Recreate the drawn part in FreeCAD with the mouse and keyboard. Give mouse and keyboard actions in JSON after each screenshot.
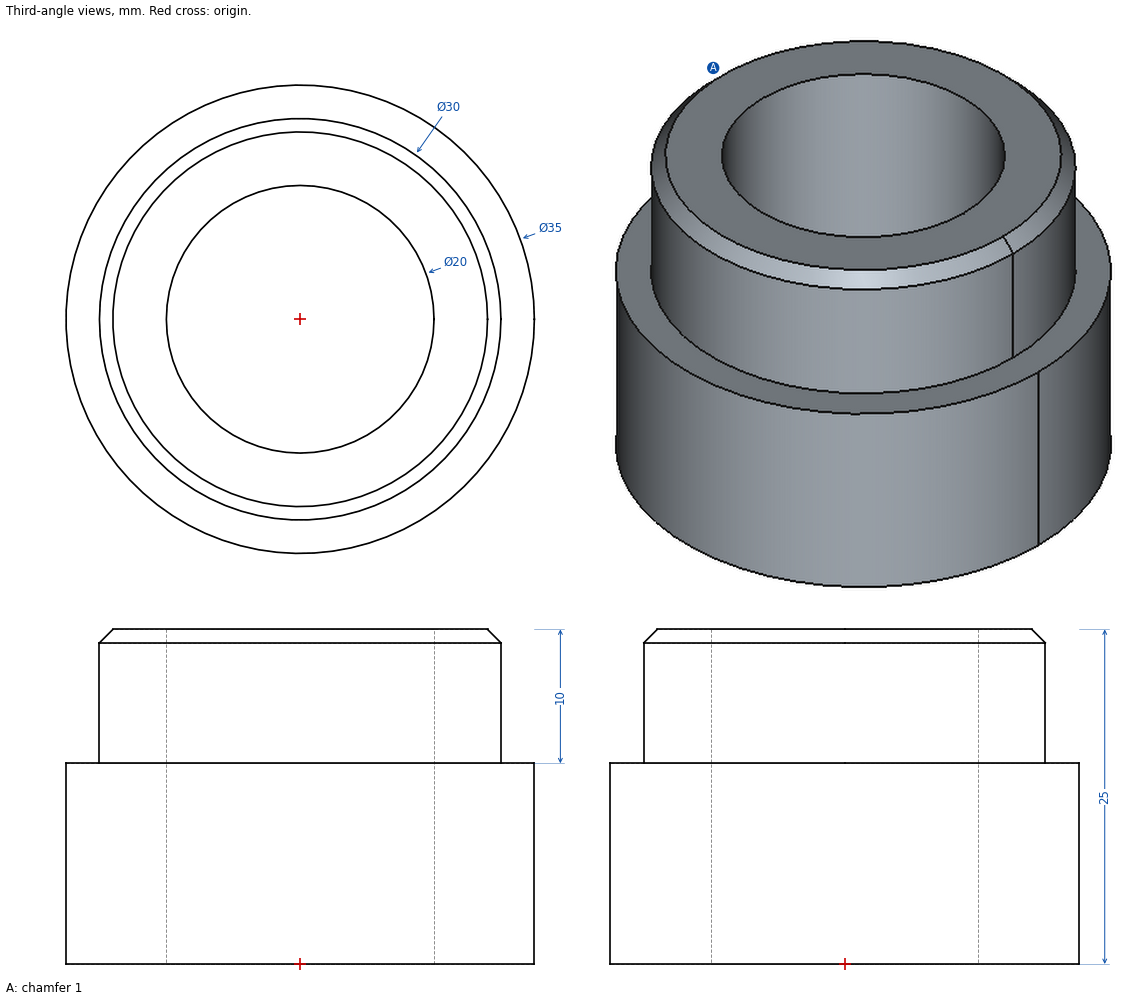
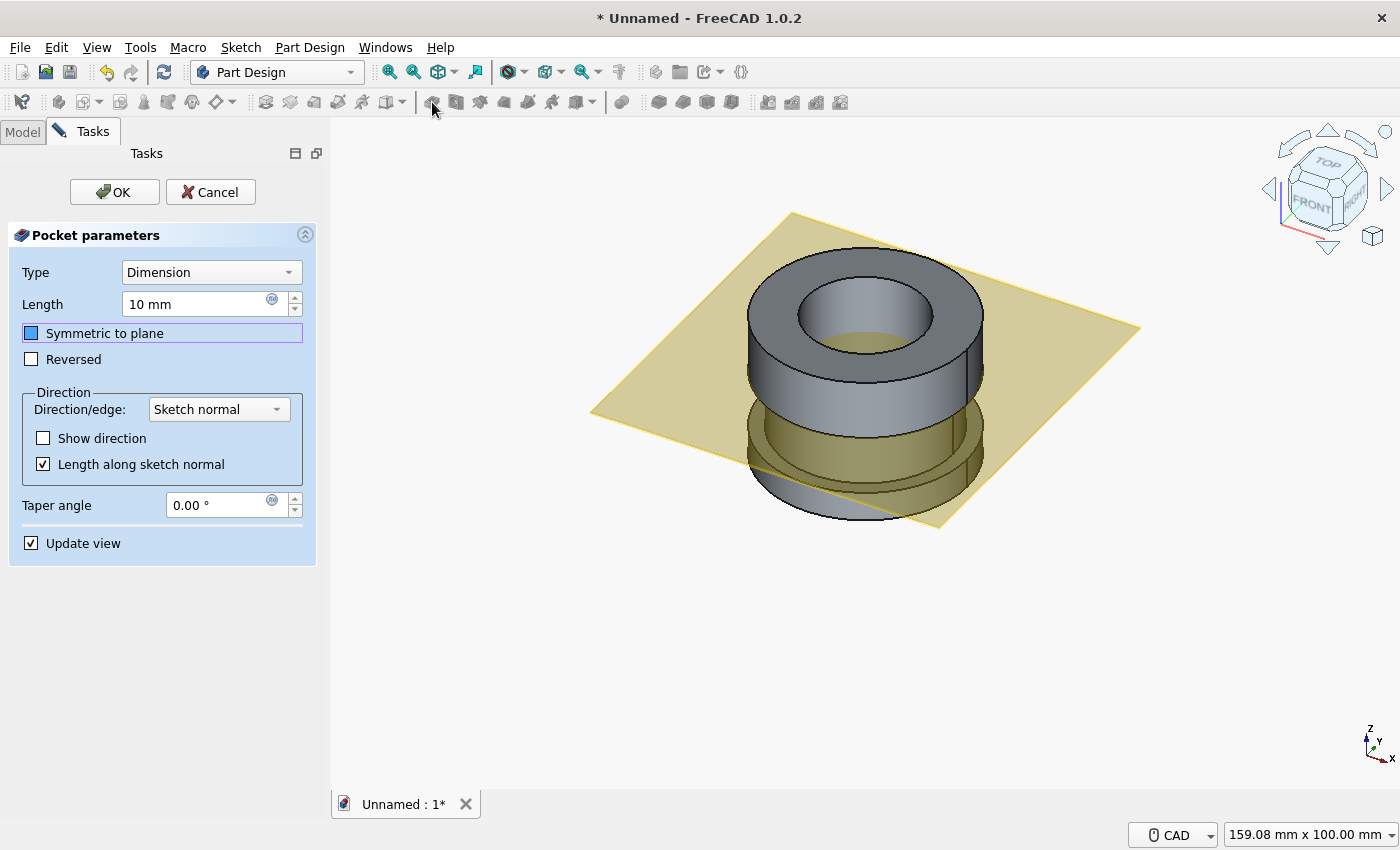
{"action": "left_click", "coordinate": [30, 359]}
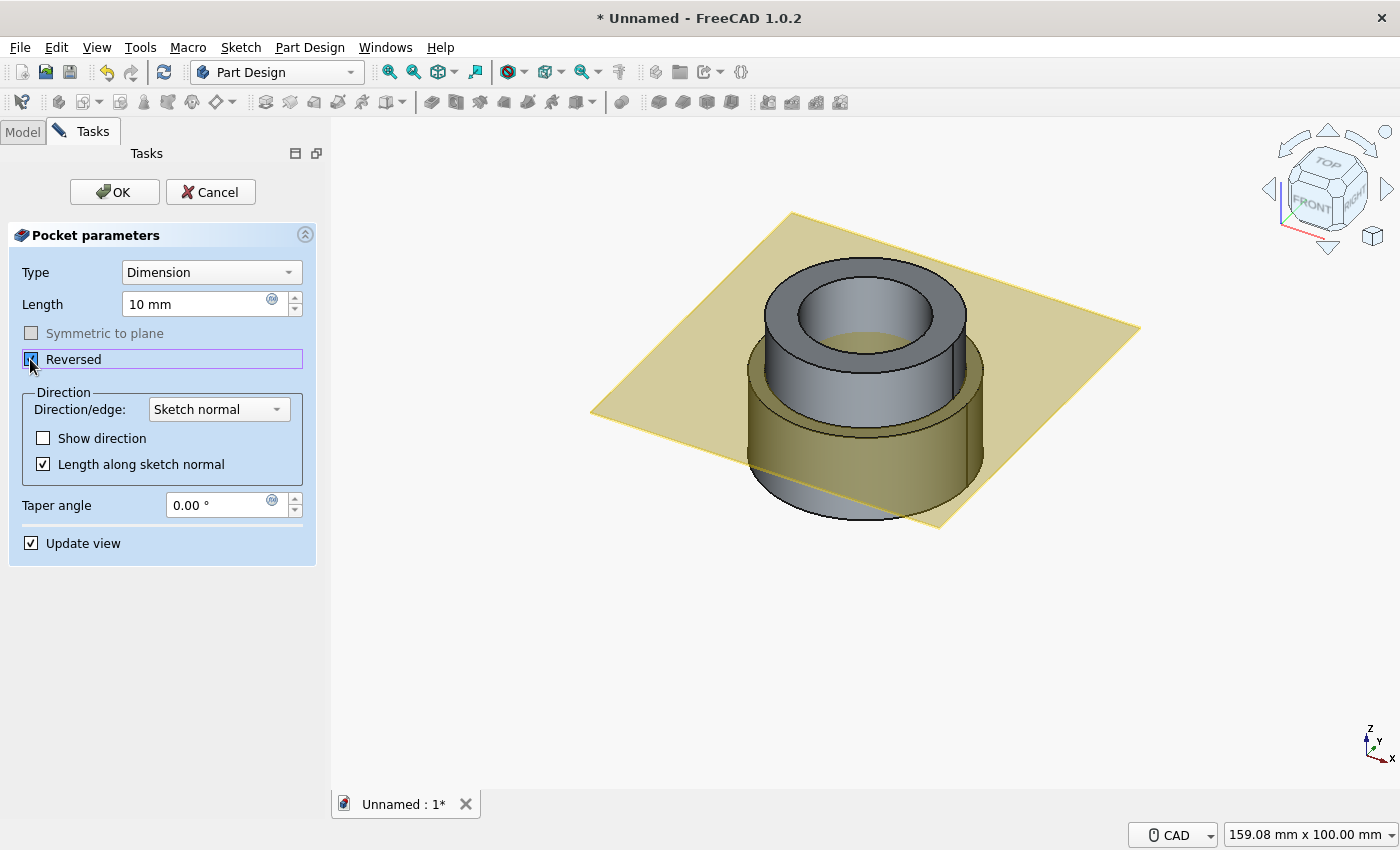
{"action": "left_click", "coordinate": [115, 192]}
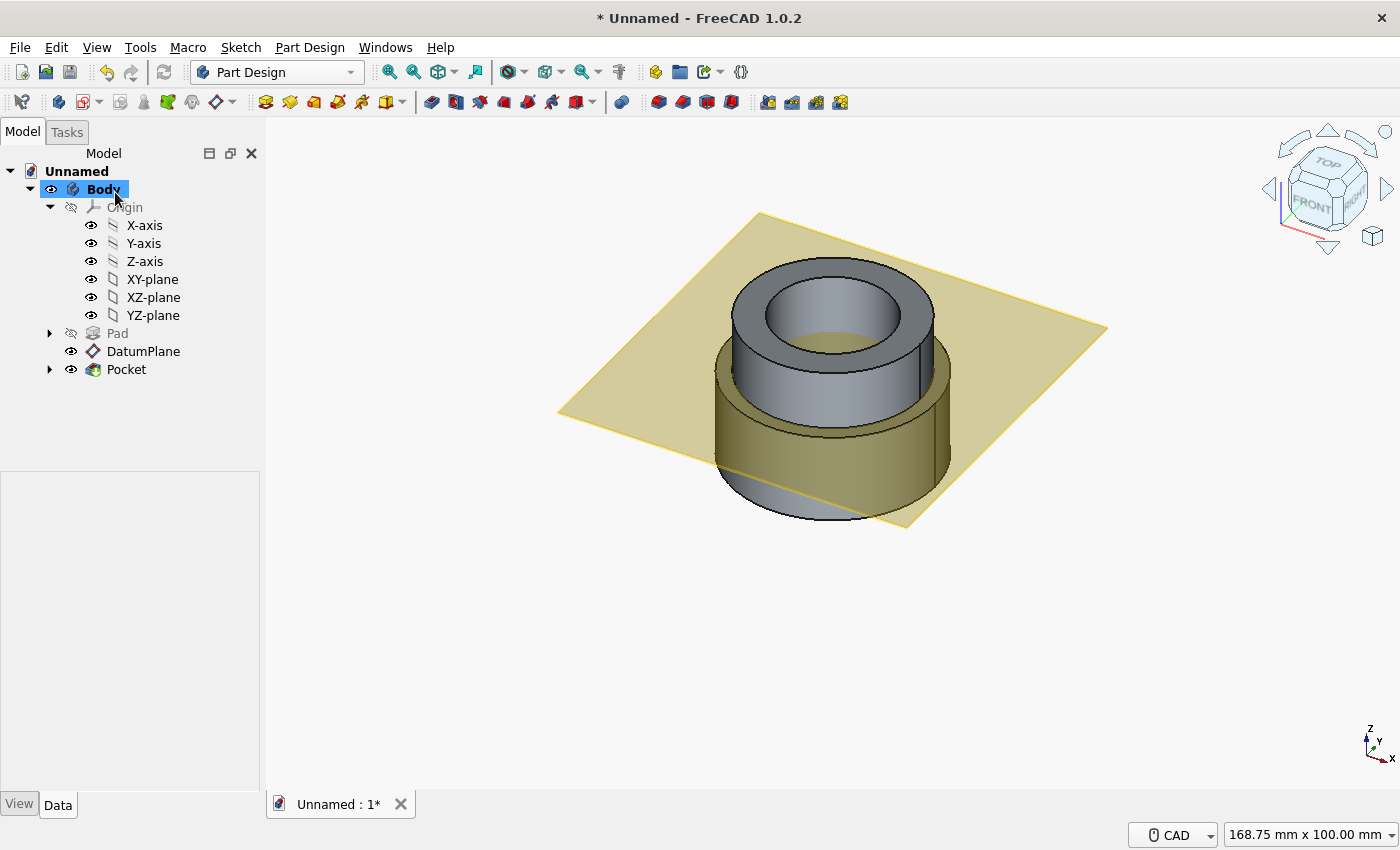
{"action": "left_click", "coordinate": [116, 351]}
{"action": "key", "text": "space"}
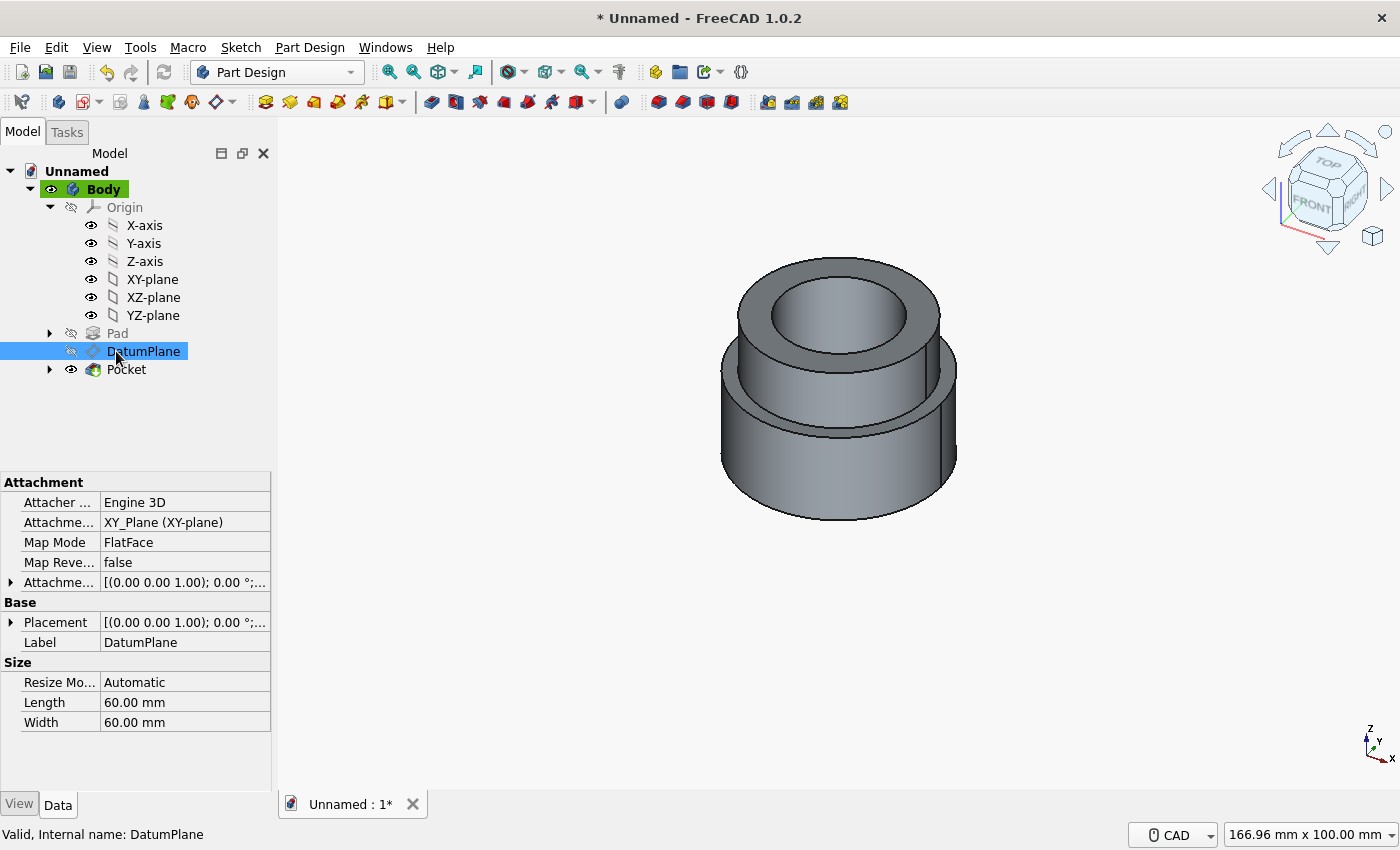
{"action": "left_click", "coordinate": [739, 320]}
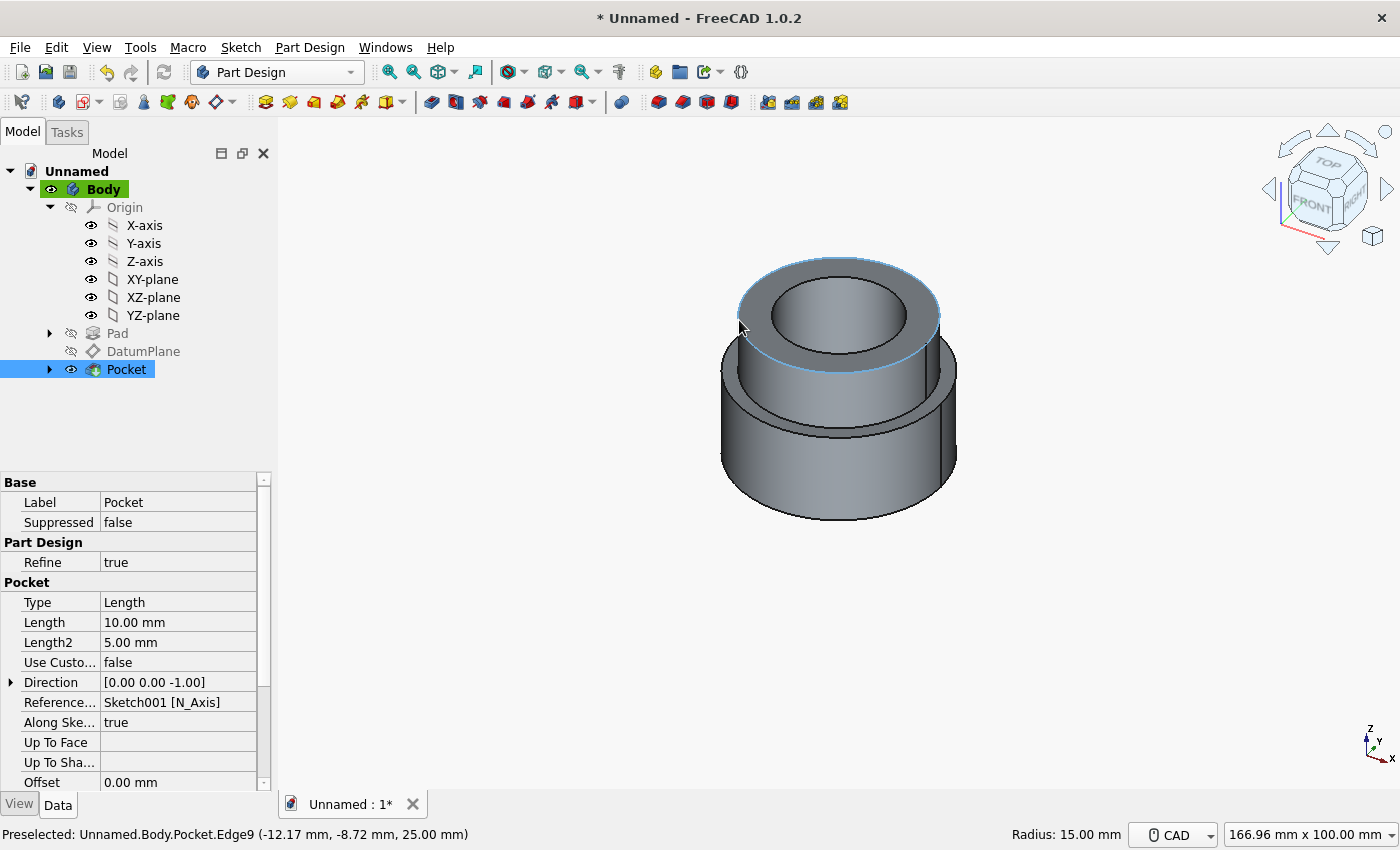
{"action": "left_click", "coordinate": [684, 102]}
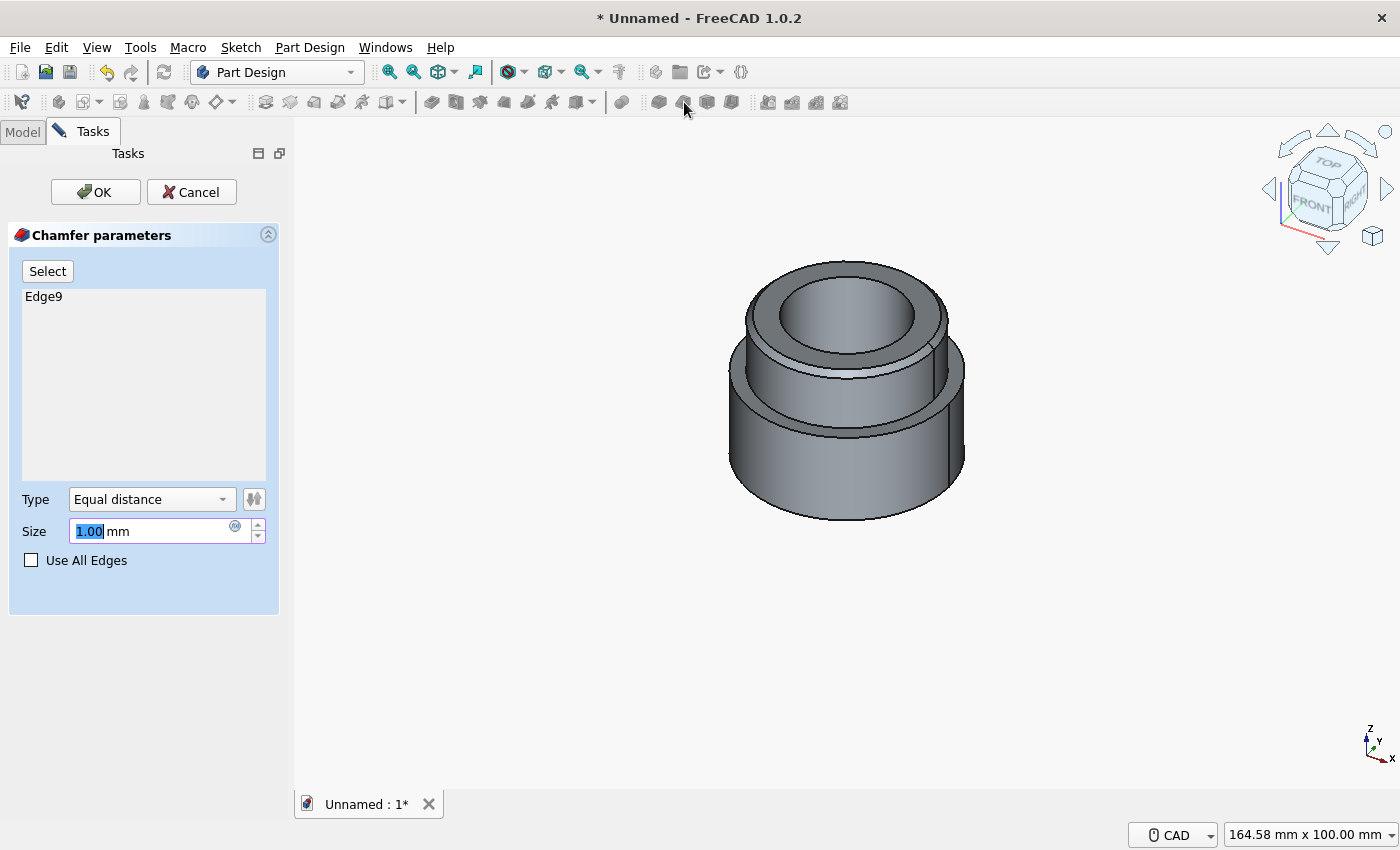
{"action": "type", "text": "1"}
{"action": "key", "text": "Tab"}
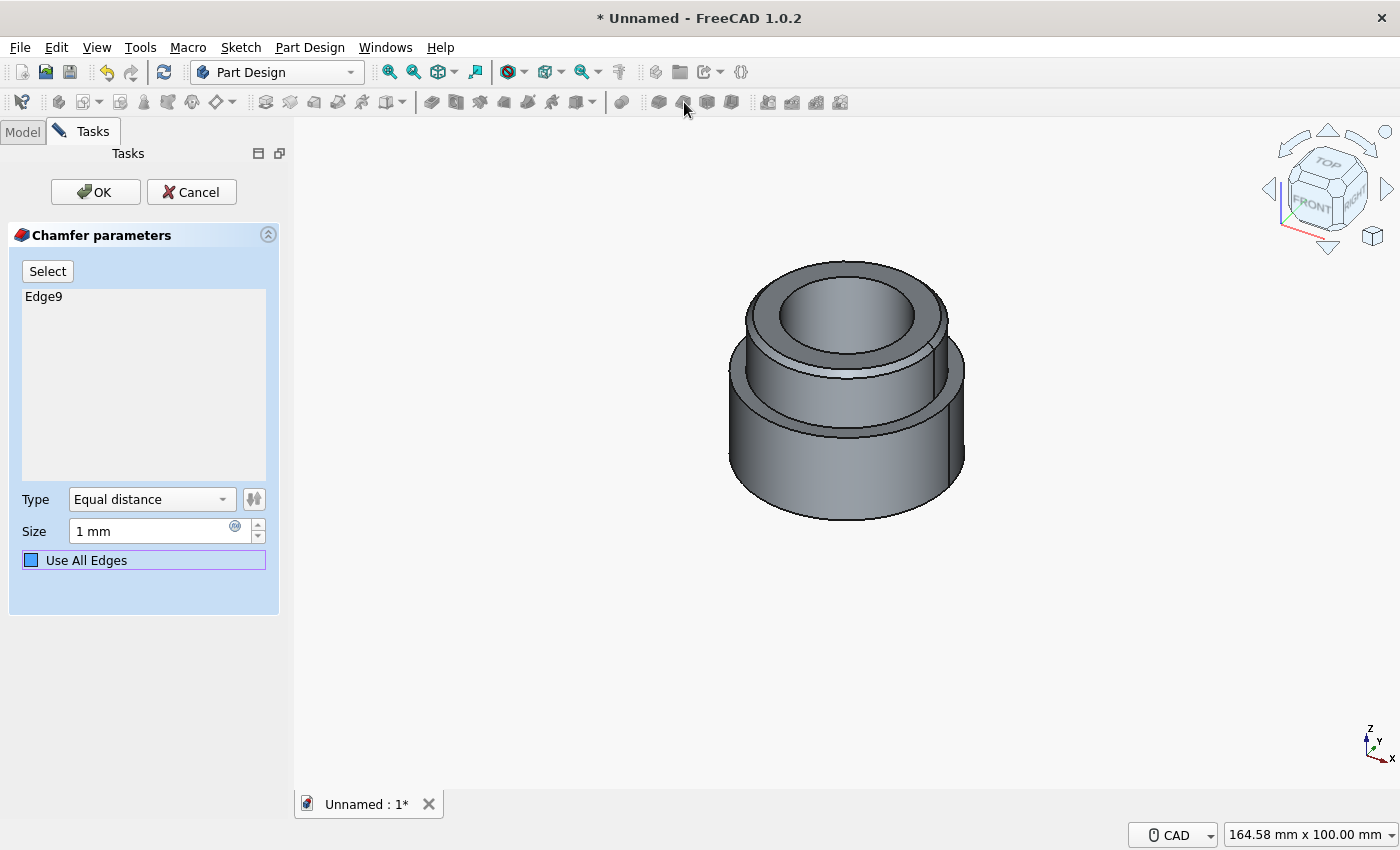
{"action": "left_click", "coordinate": [96, 192]}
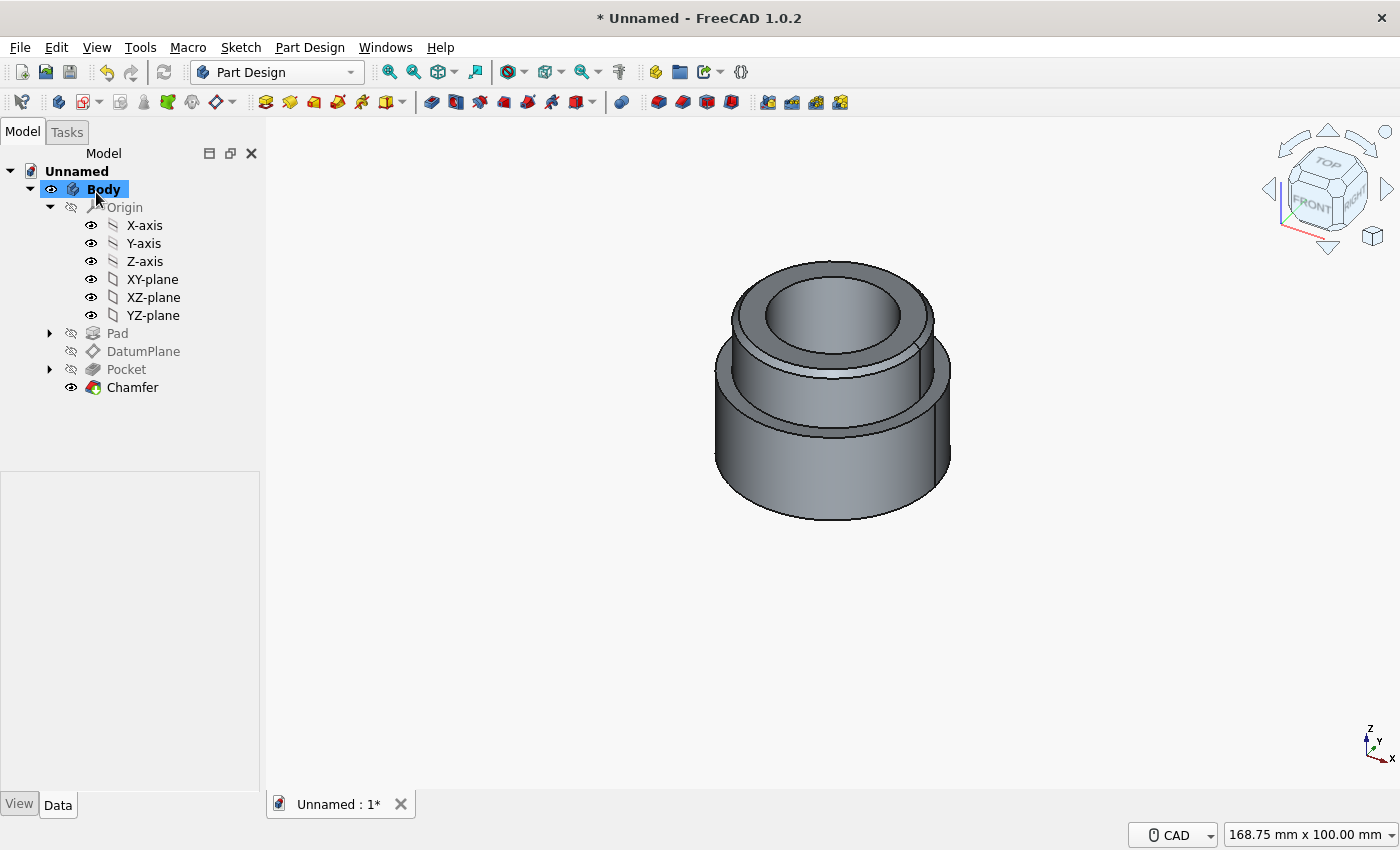
{"action": "key", "text": "0"}